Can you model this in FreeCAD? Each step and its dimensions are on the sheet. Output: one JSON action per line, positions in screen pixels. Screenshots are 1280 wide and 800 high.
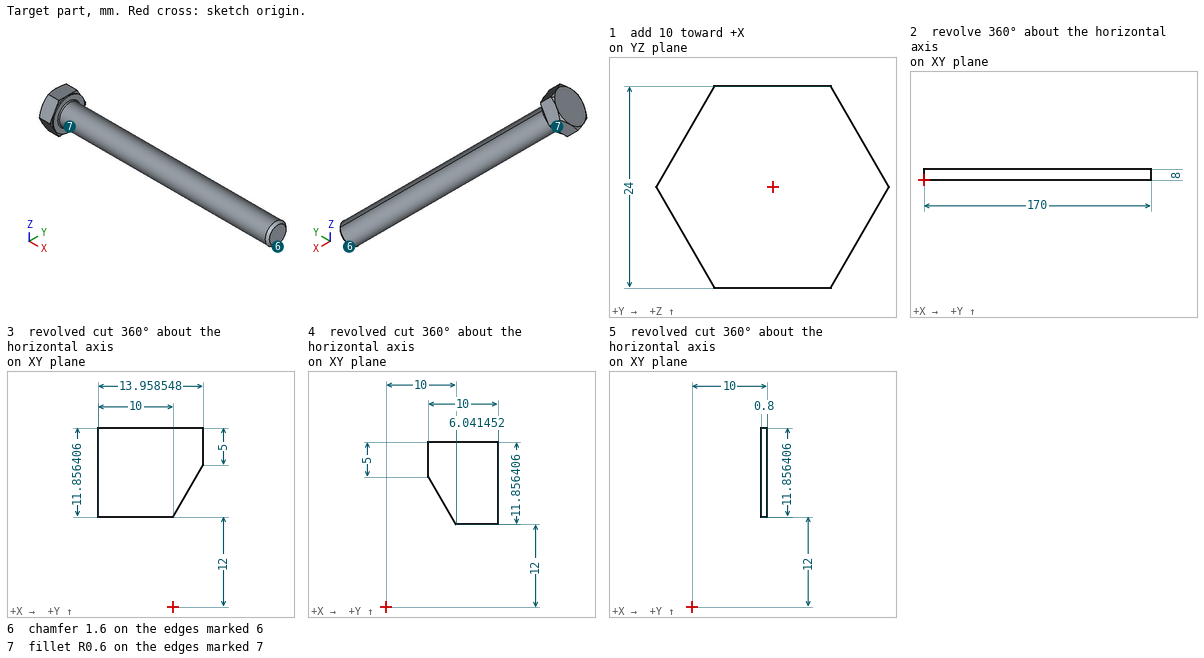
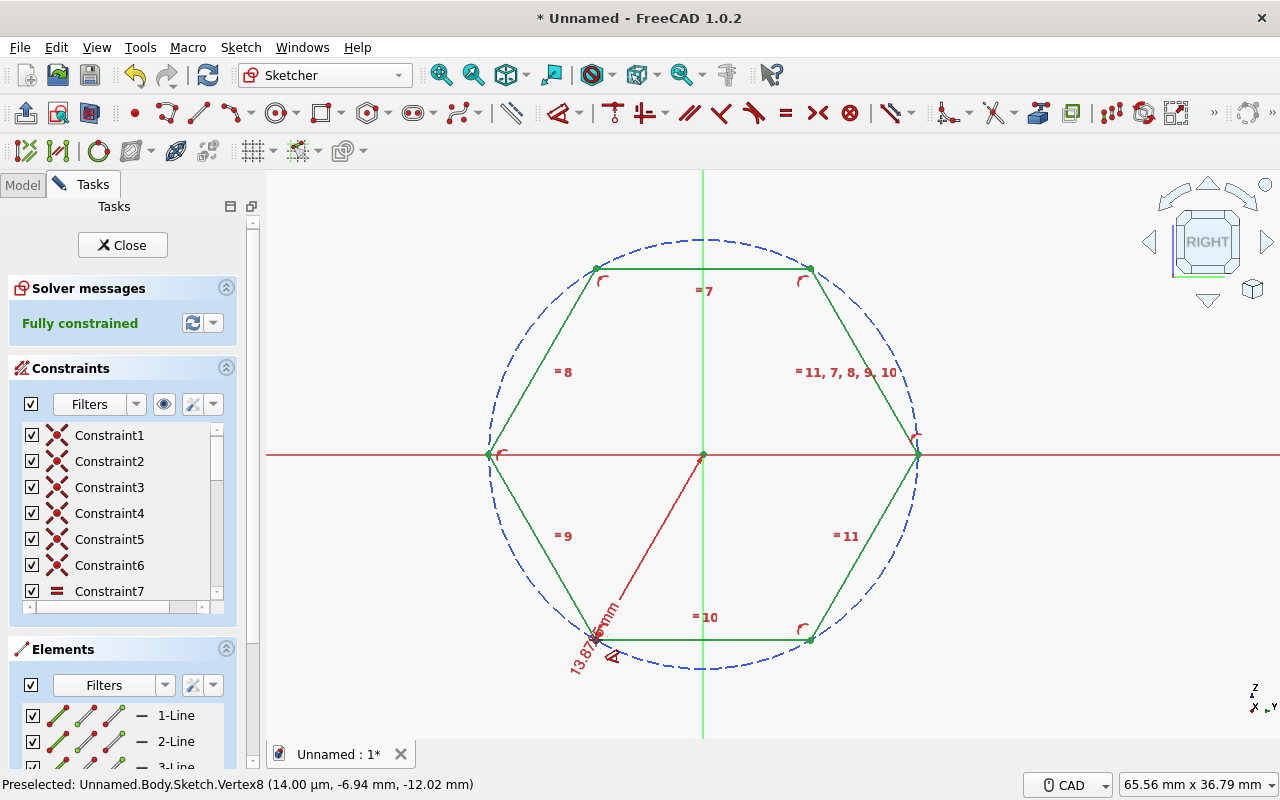
{"action": "left_click", "coordinate": [811, 269]}
{"action": "left_click", "coordinate": [562, 369]}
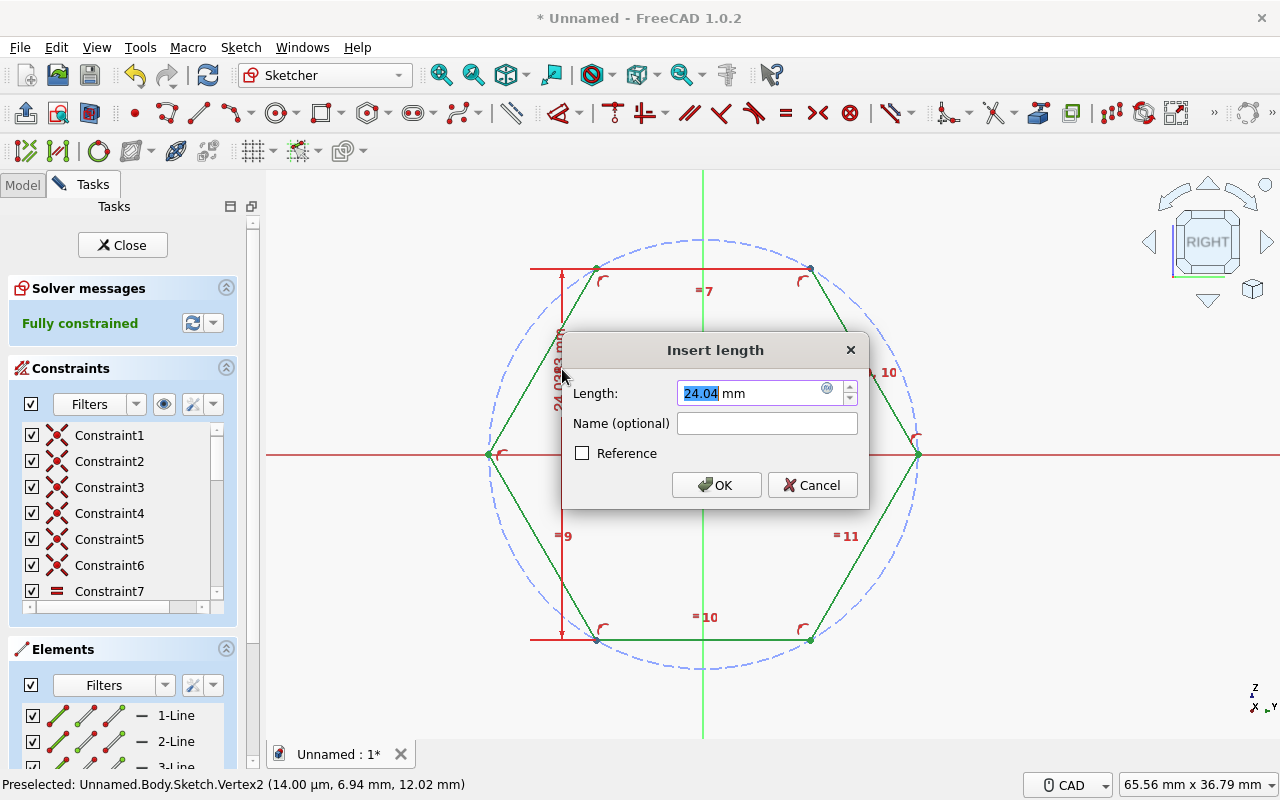
{"action": "type", "text": "24"}
{"action": "key", "text": "Return"}
{"action": "key", "text": "Escape"}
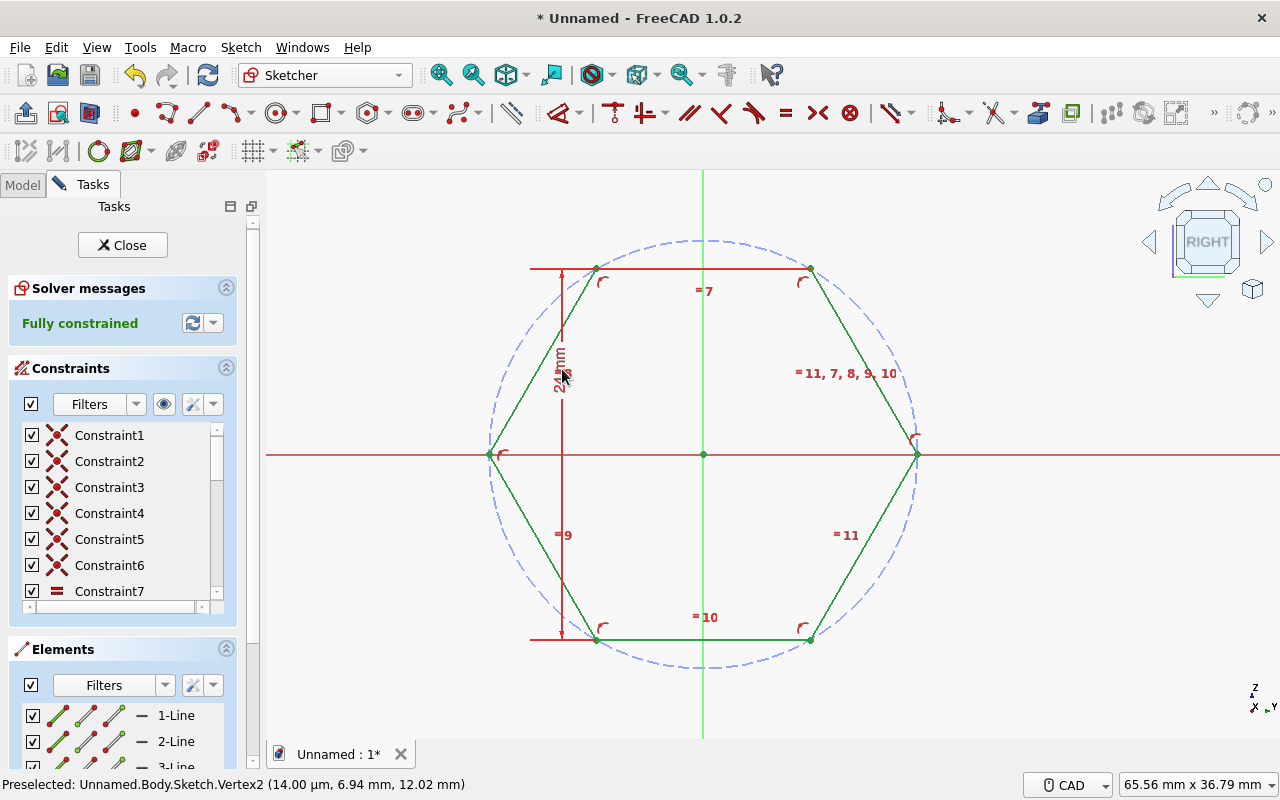
{"action": "left_click", "coordinate": [123, 245]}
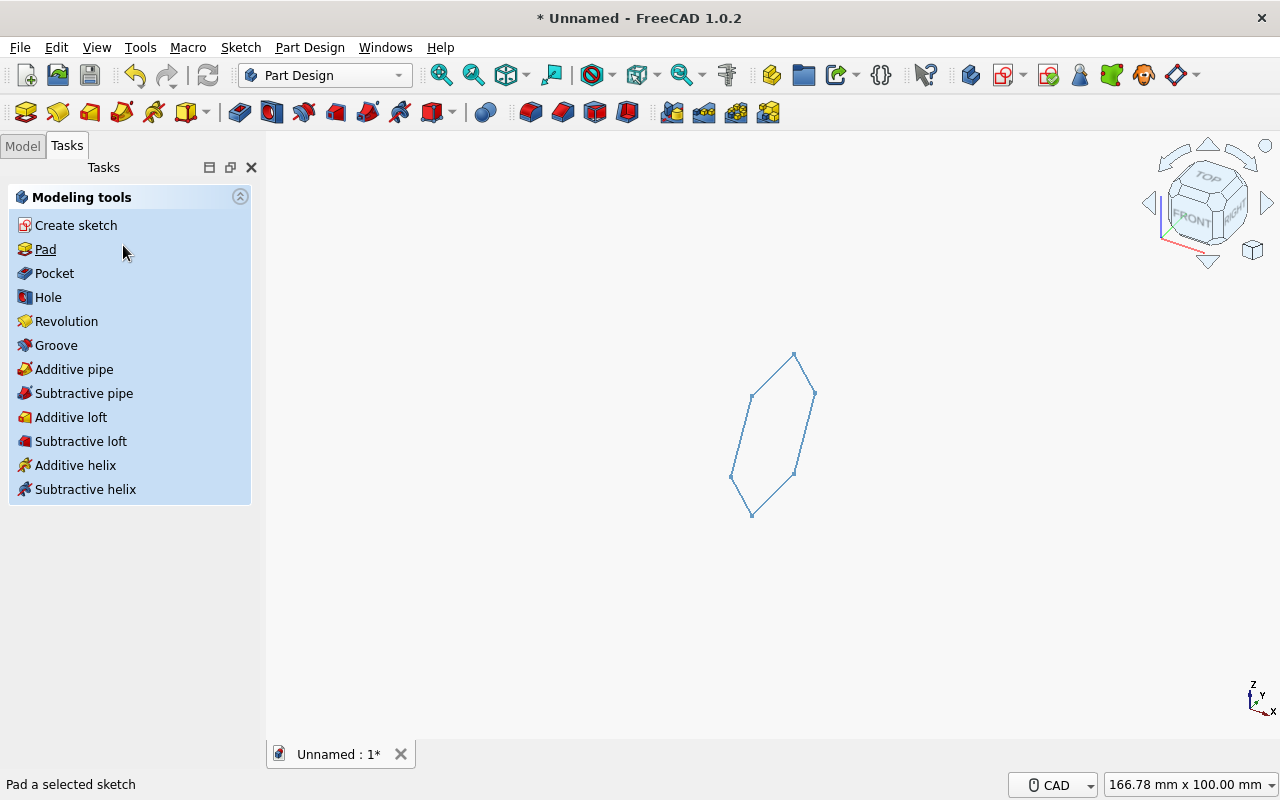
{"action": "left_click", "coordinate": [26, 112]}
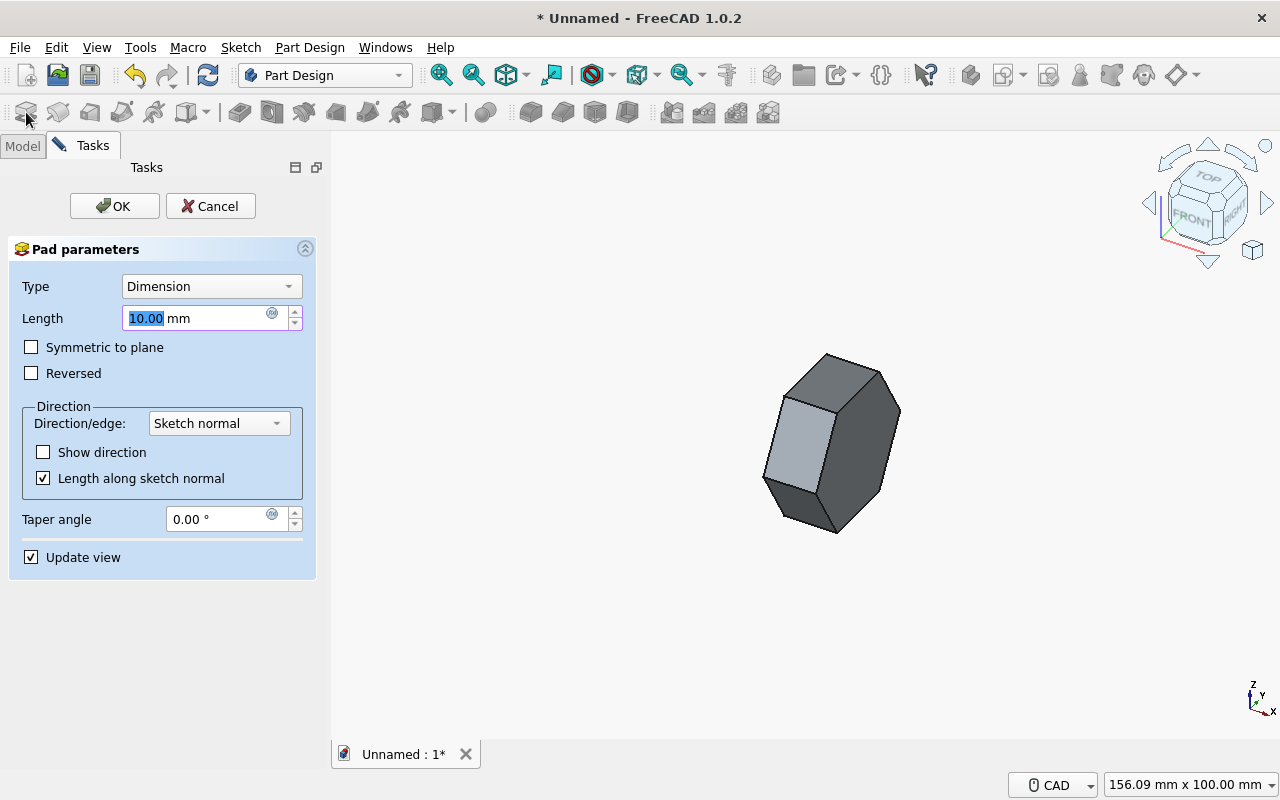
{"action": "type", "text": "10"}
{"action": "key", "text": "Tab"}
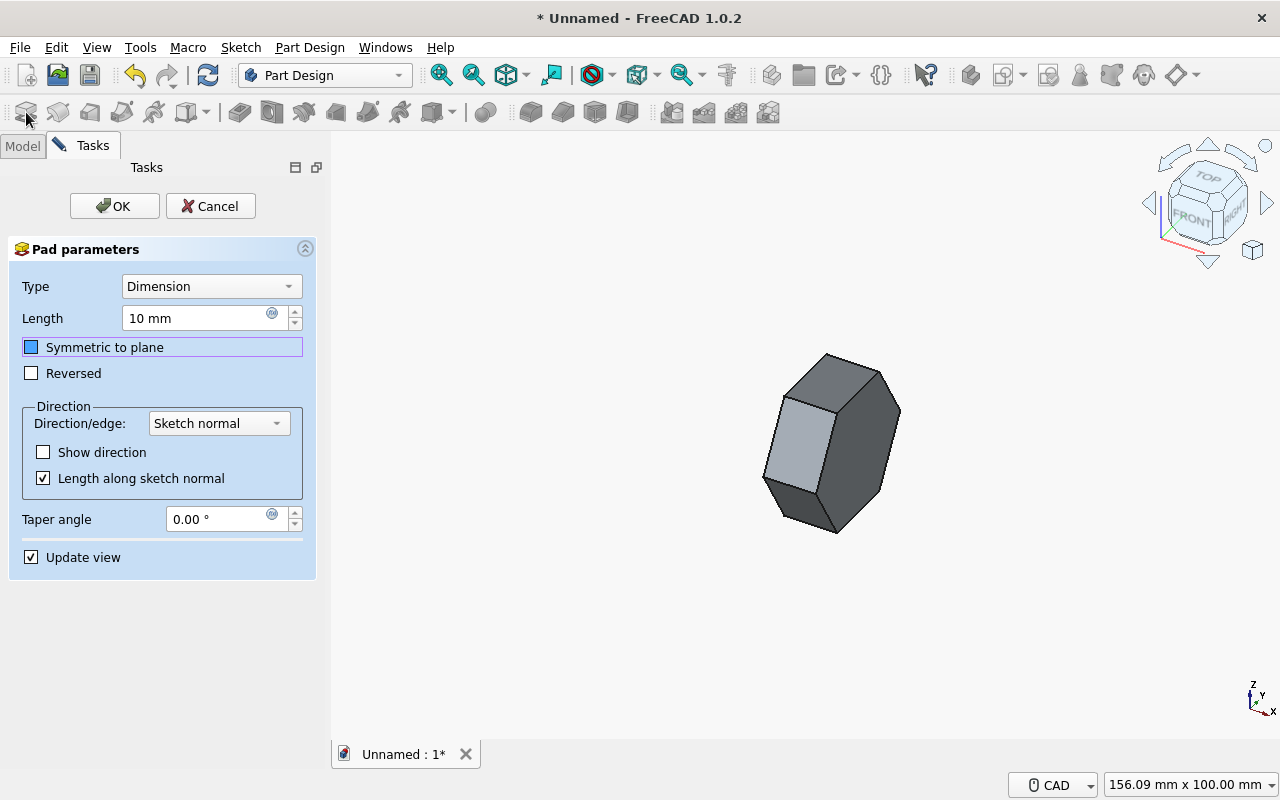
{"action": "left_click", "coordinate": [115, 206]}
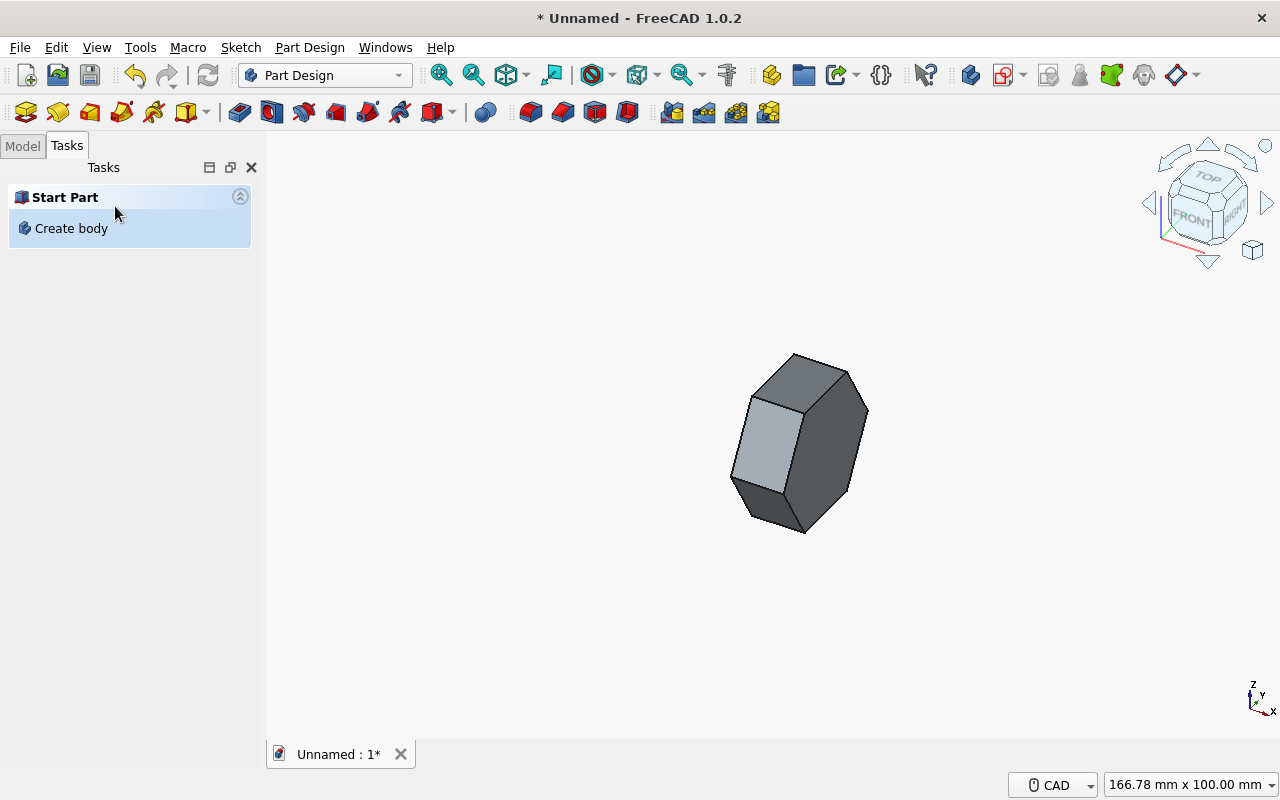
{"action": "left_click", "coordinate": [442, 76]}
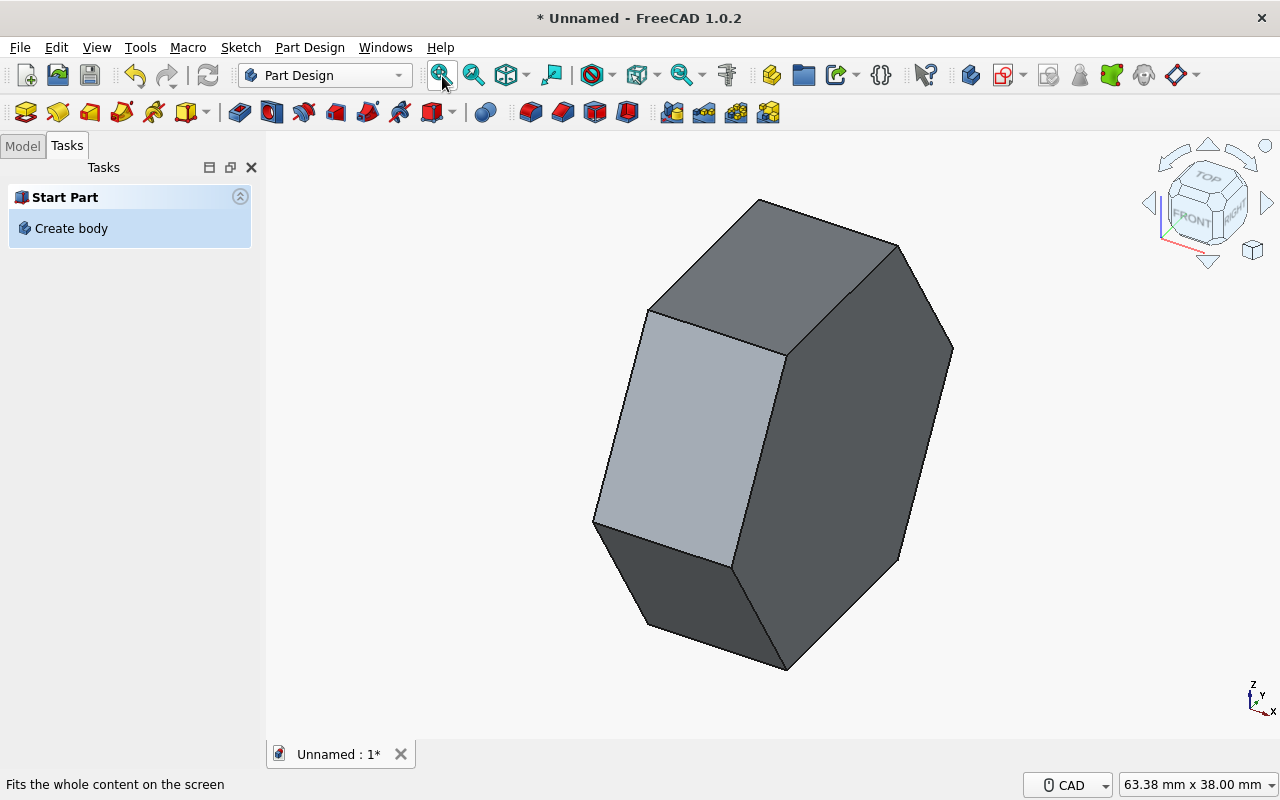
{"action": "left_click", "coordinate": [1004, 76]}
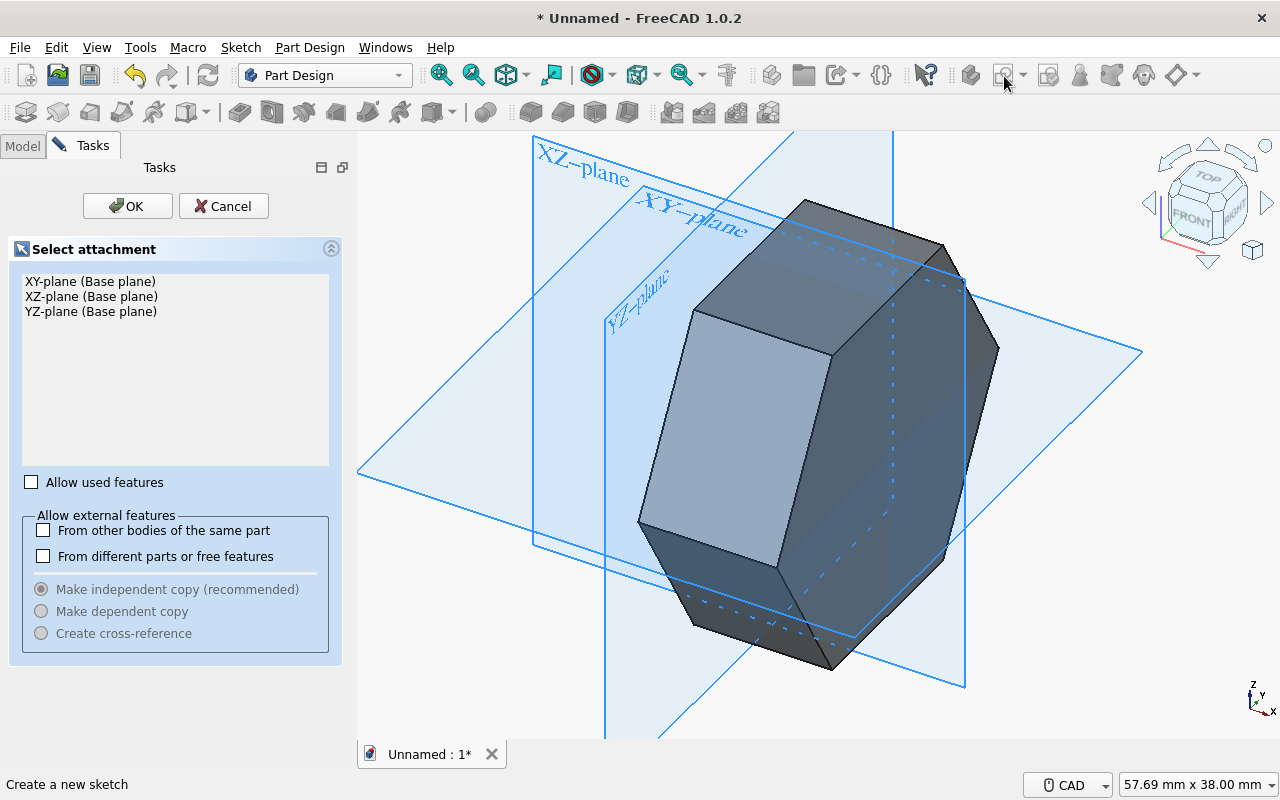
{"action": "left_click", "coordinate": [82, 282]}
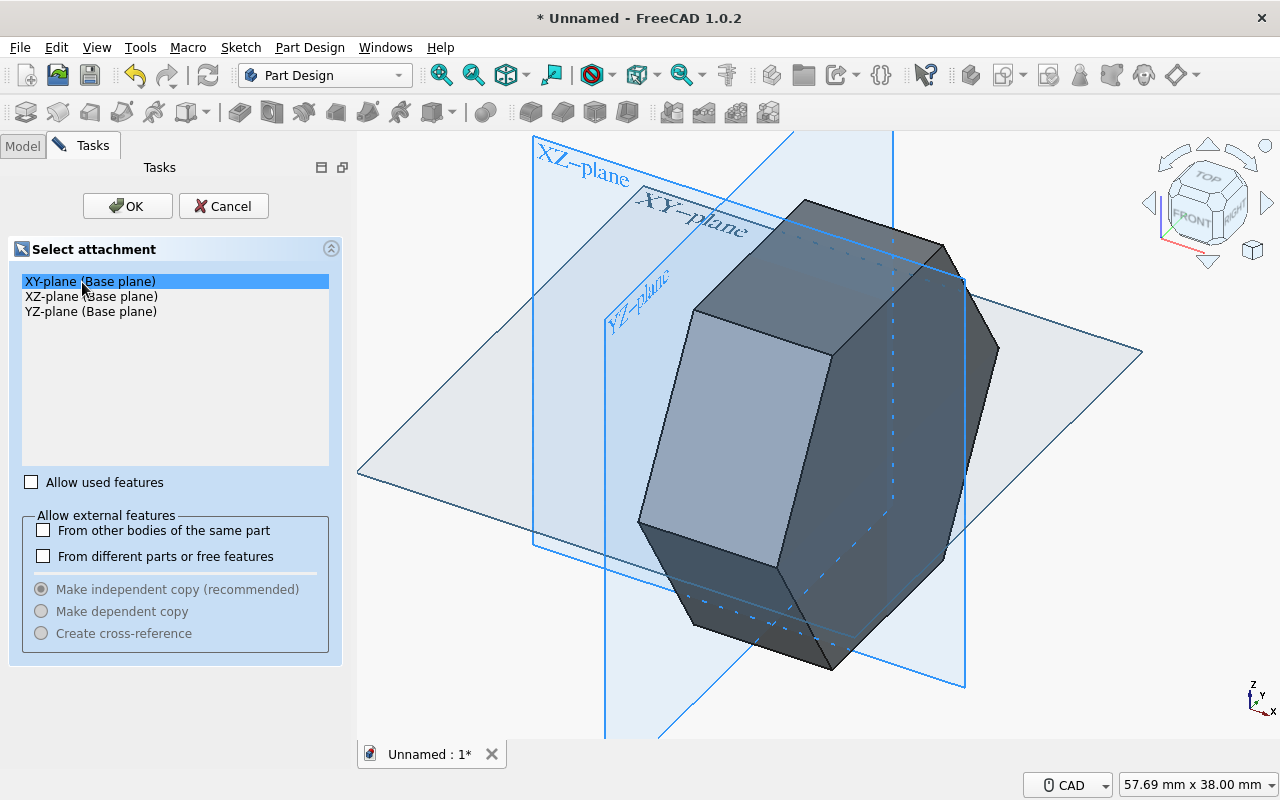
{"action": "left_click", "coordinate": [128, 206]}